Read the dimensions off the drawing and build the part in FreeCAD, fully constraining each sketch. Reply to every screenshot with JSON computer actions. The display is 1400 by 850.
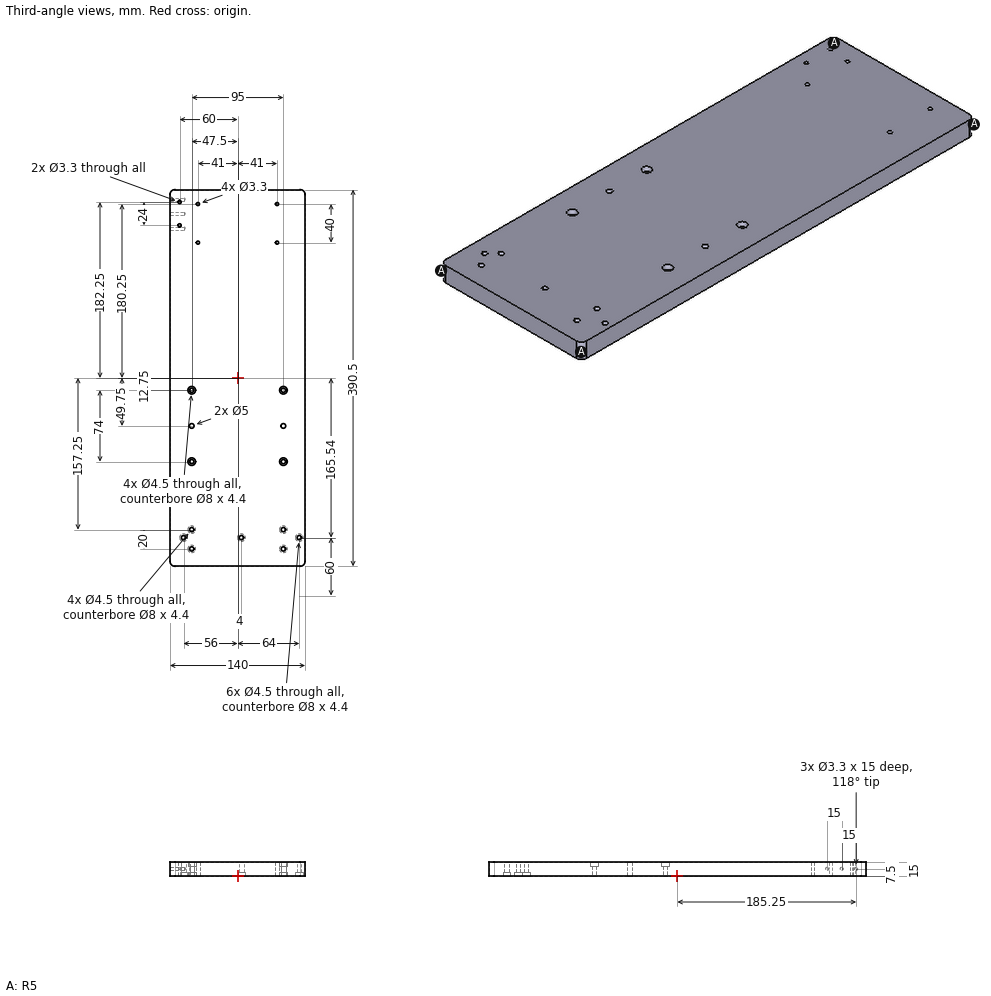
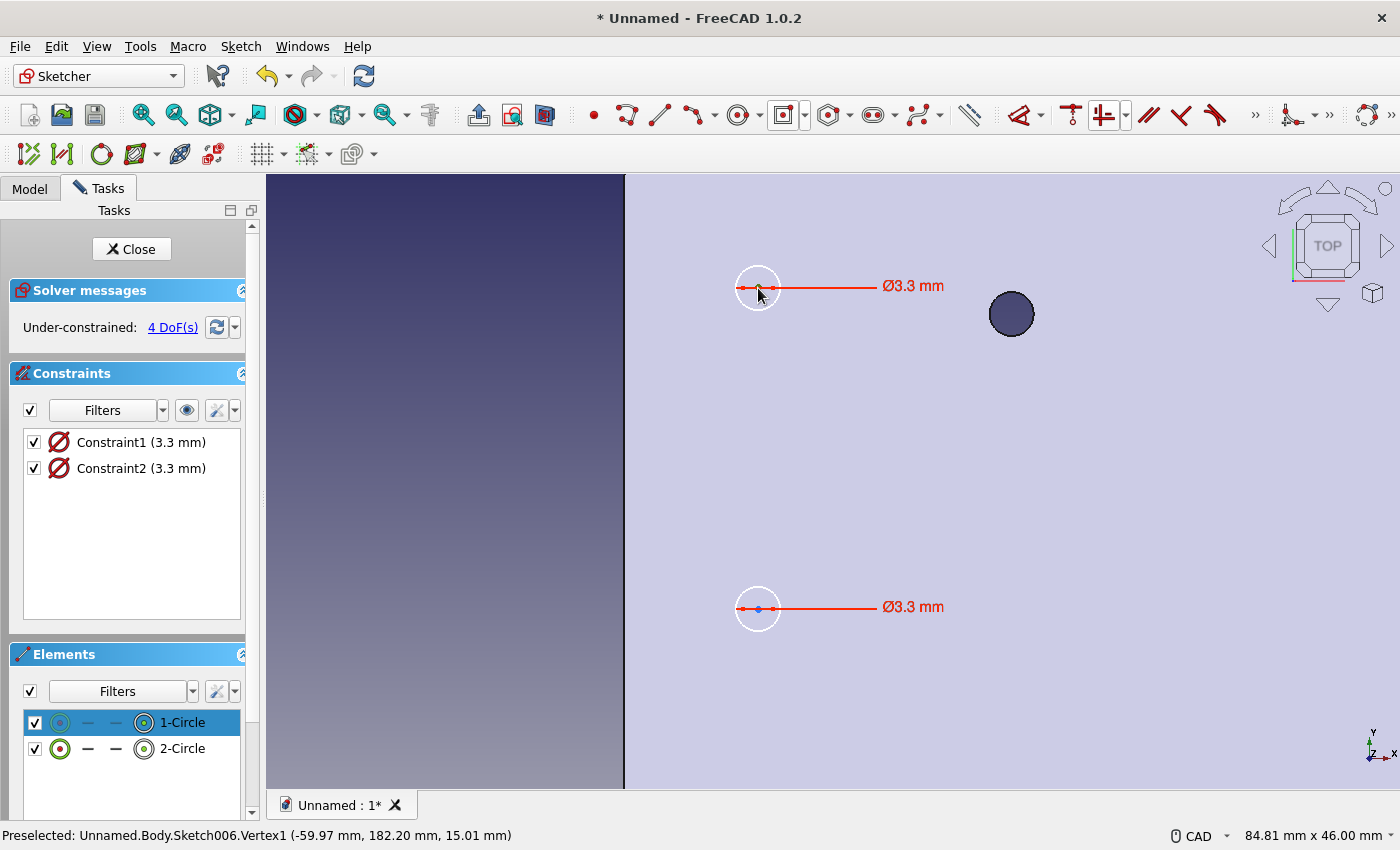
{"action": "left_click", "coordinate": [758, 609]}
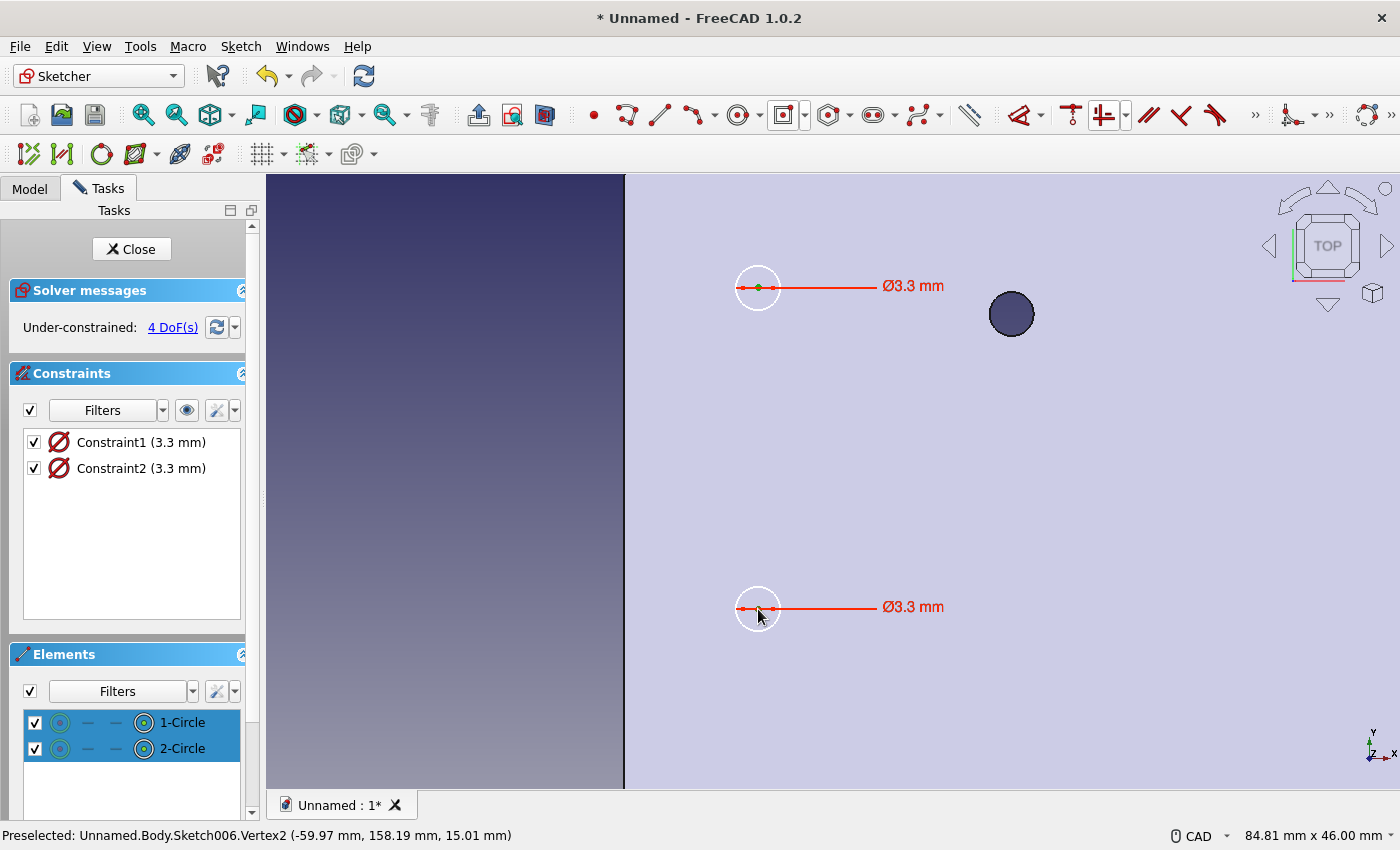
{"action": "key", "text": "v"}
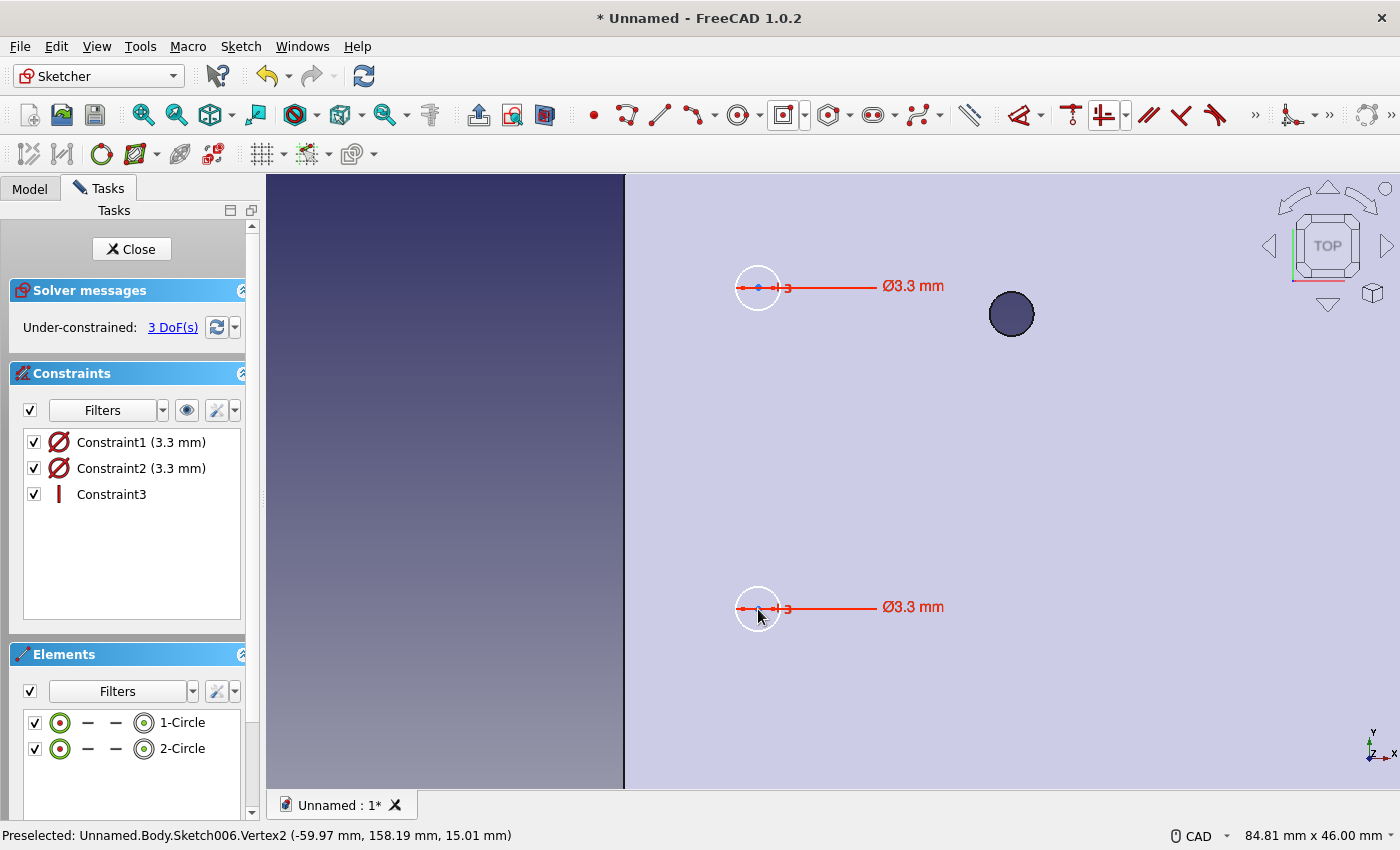
{"action": "left_click", "coordinate": [1018, 116]}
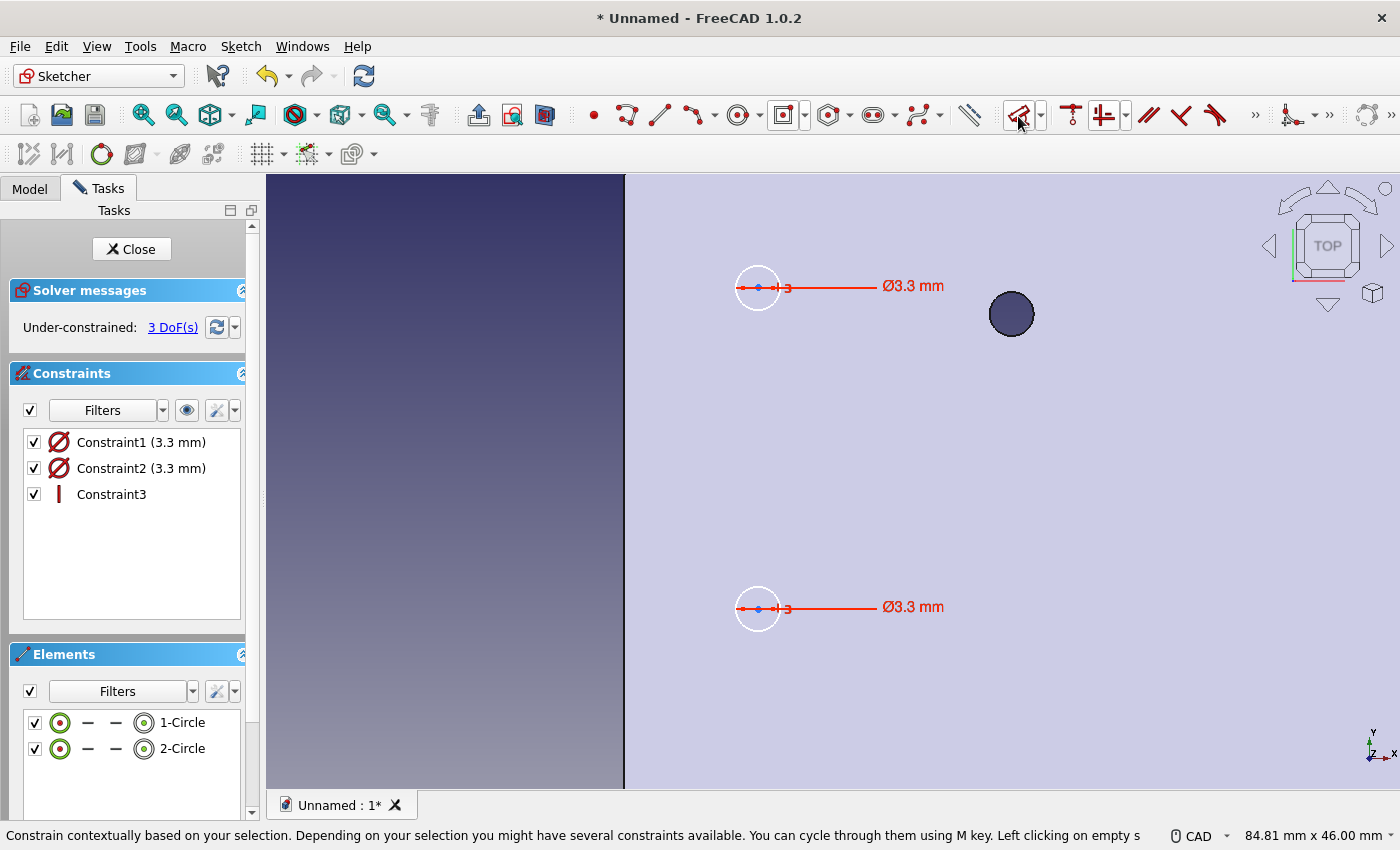
{"action": "left_click", "coordinate": [758, 288]}
{"action": "left_click", "coordinate": [996, 254]}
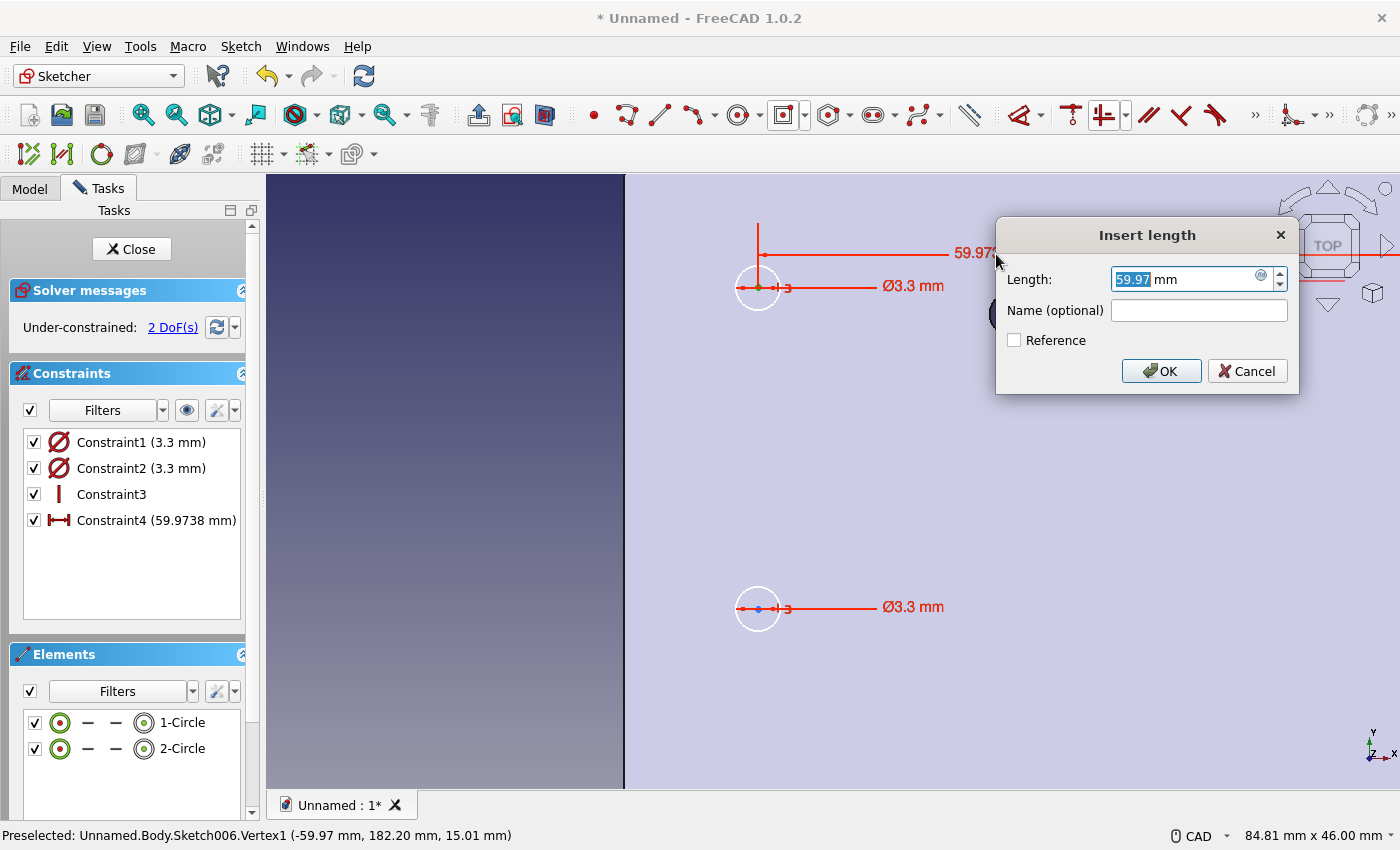
{"action": "type", "text": "60"}
{"action": "key", "text": "Return"}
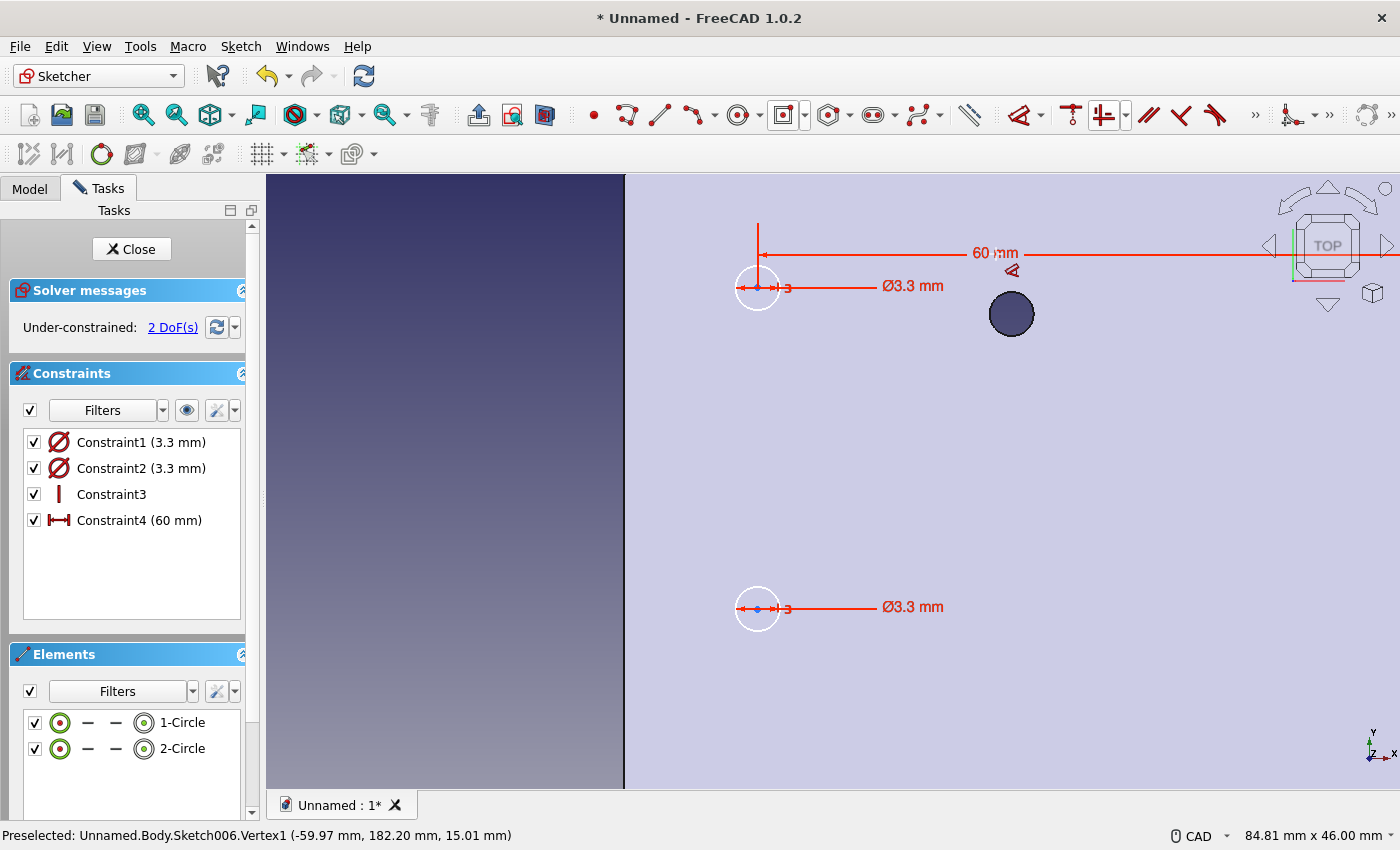
{"action": "left_click", "coordinate": [758, 288]}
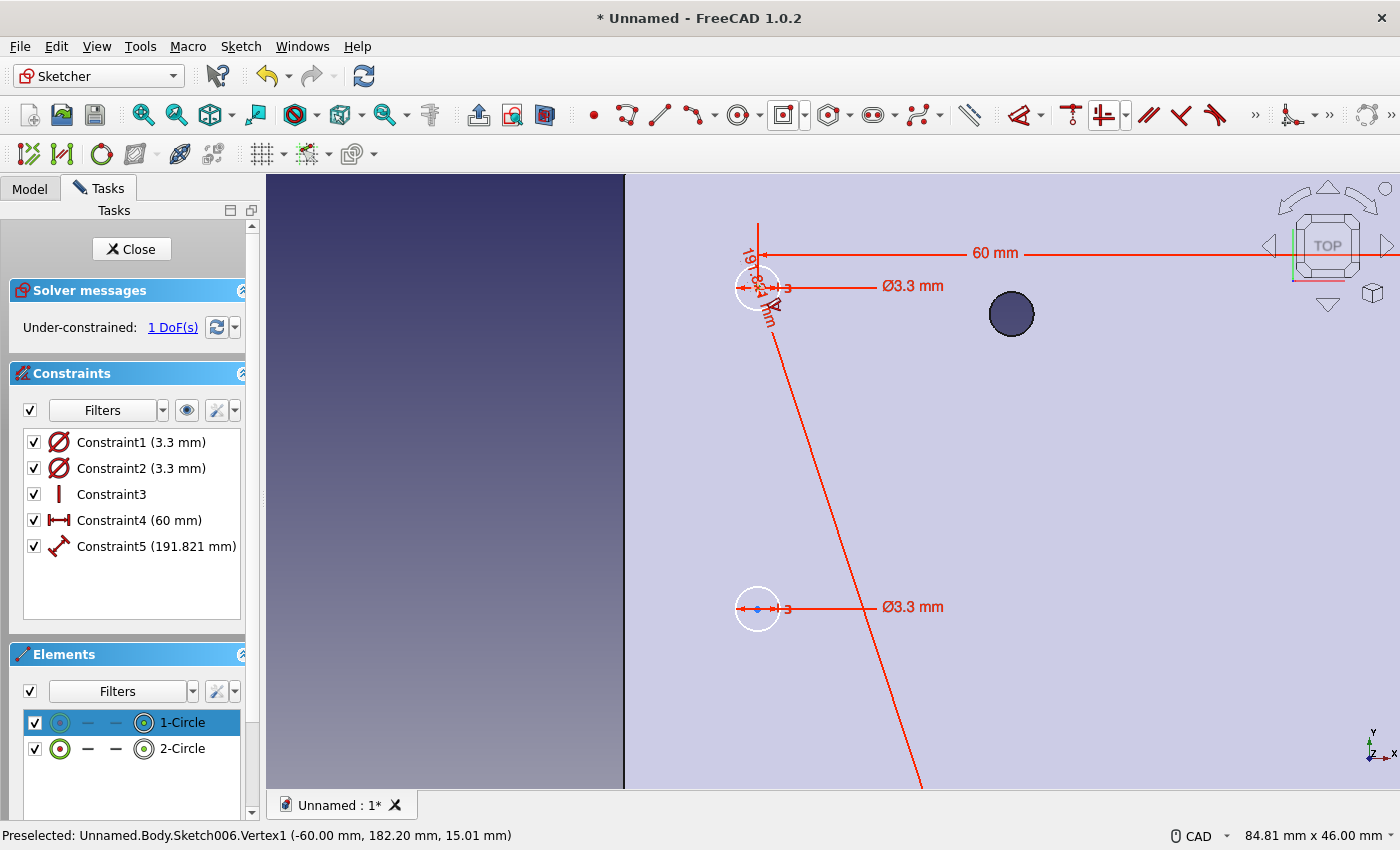
{"action": "left_click", "coordinate": [758, 609]}
{"action": "left_click", "coordinate": [792, 449]}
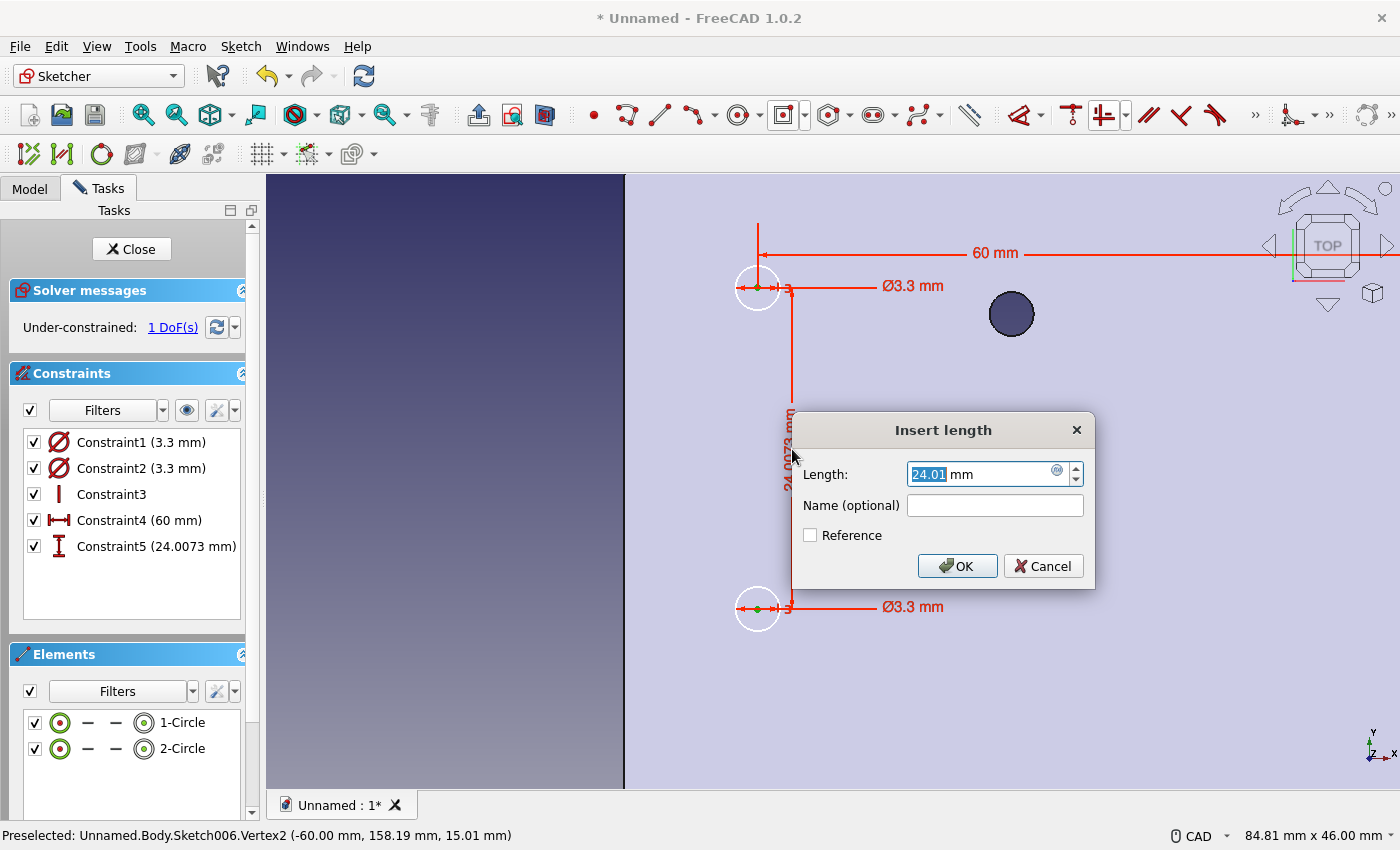
{"action": "type", "text": "24"}
{"action": "key", "text": "Return"}